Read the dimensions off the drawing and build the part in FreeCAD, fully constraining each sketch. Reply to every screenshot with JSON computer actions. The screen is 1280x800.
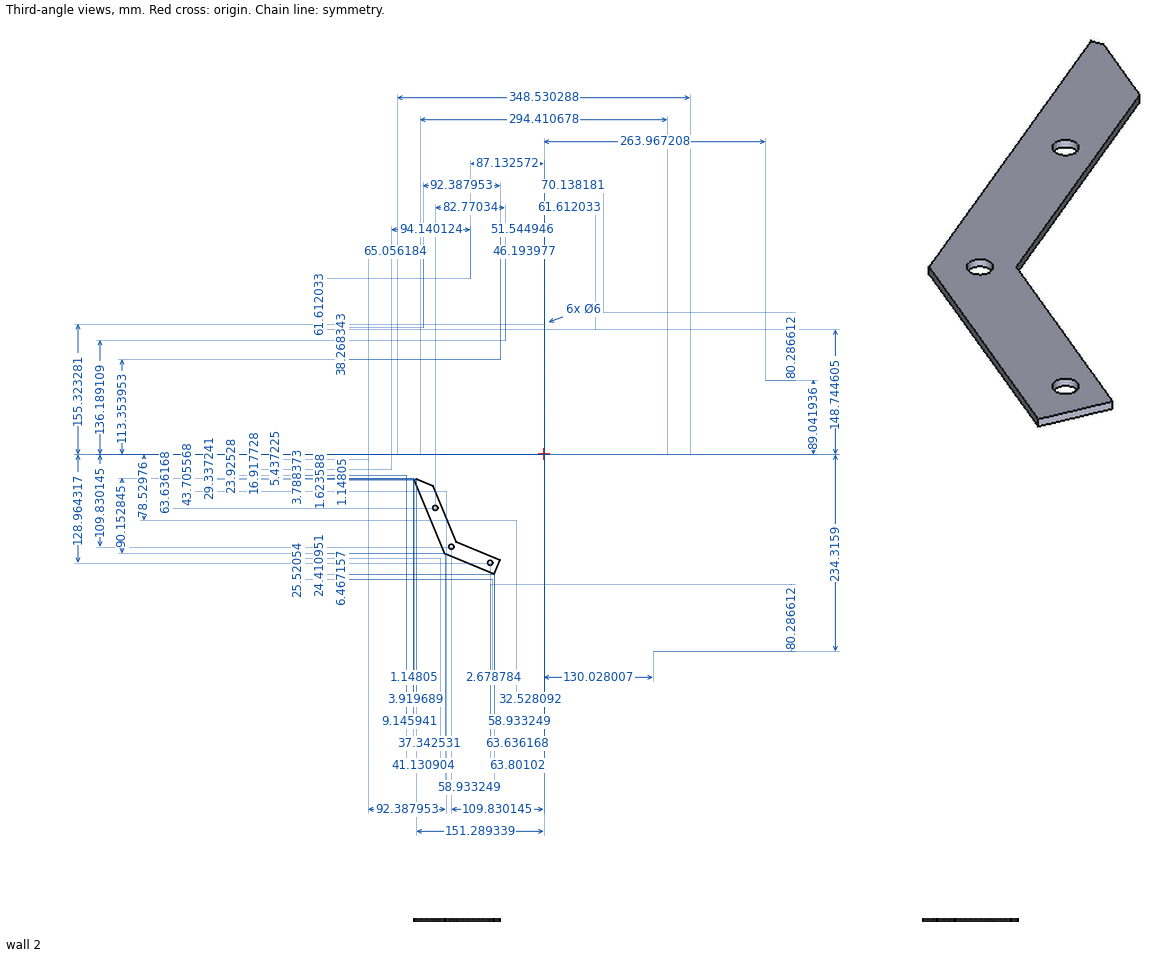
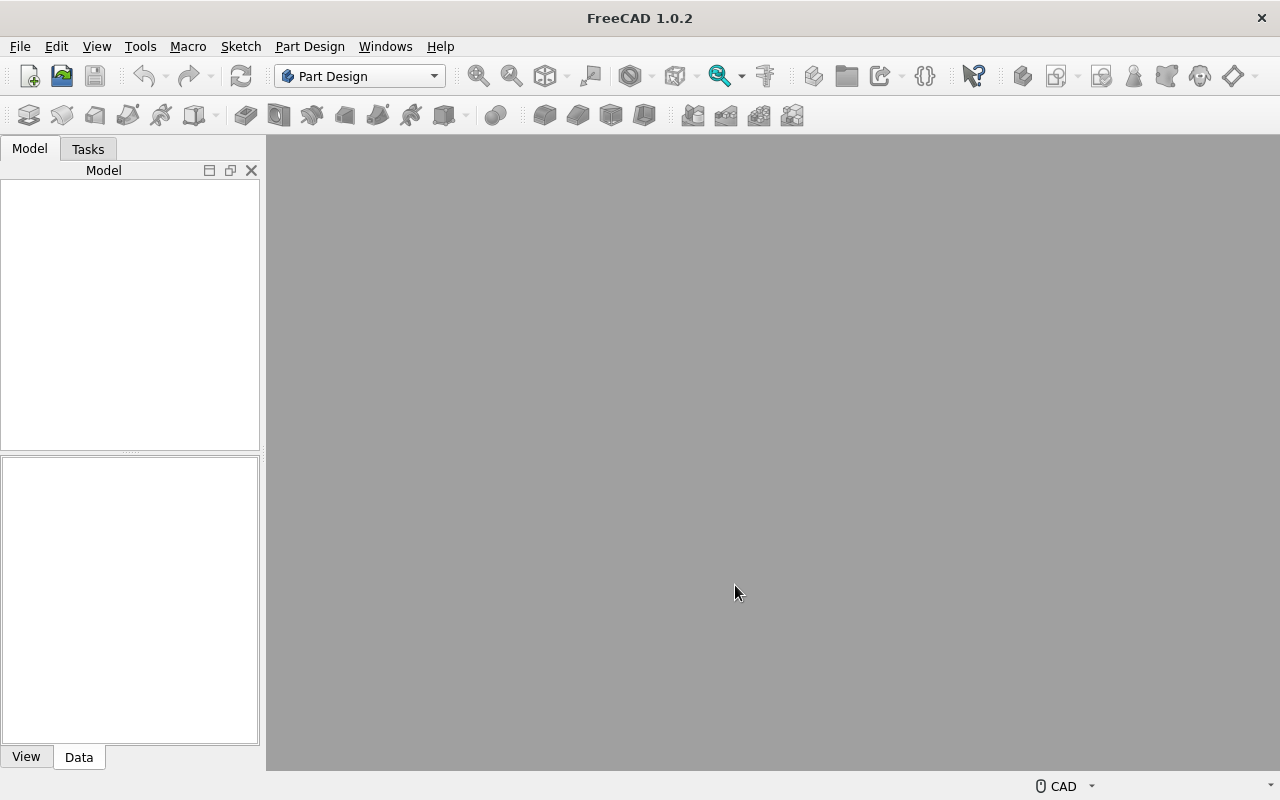
{"action": "left_click", "coordinate": [29, 76]}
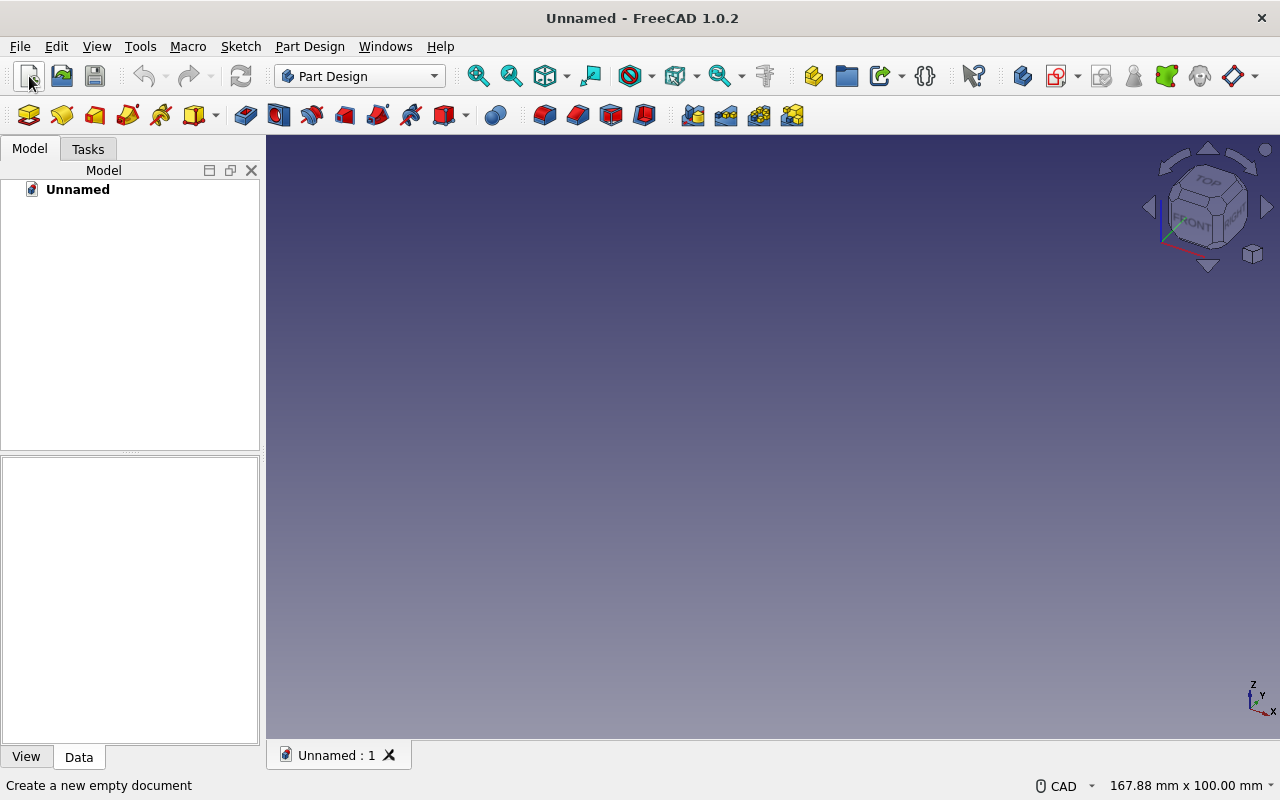
{"action": "left_click", "coordinate": [1056, 76]}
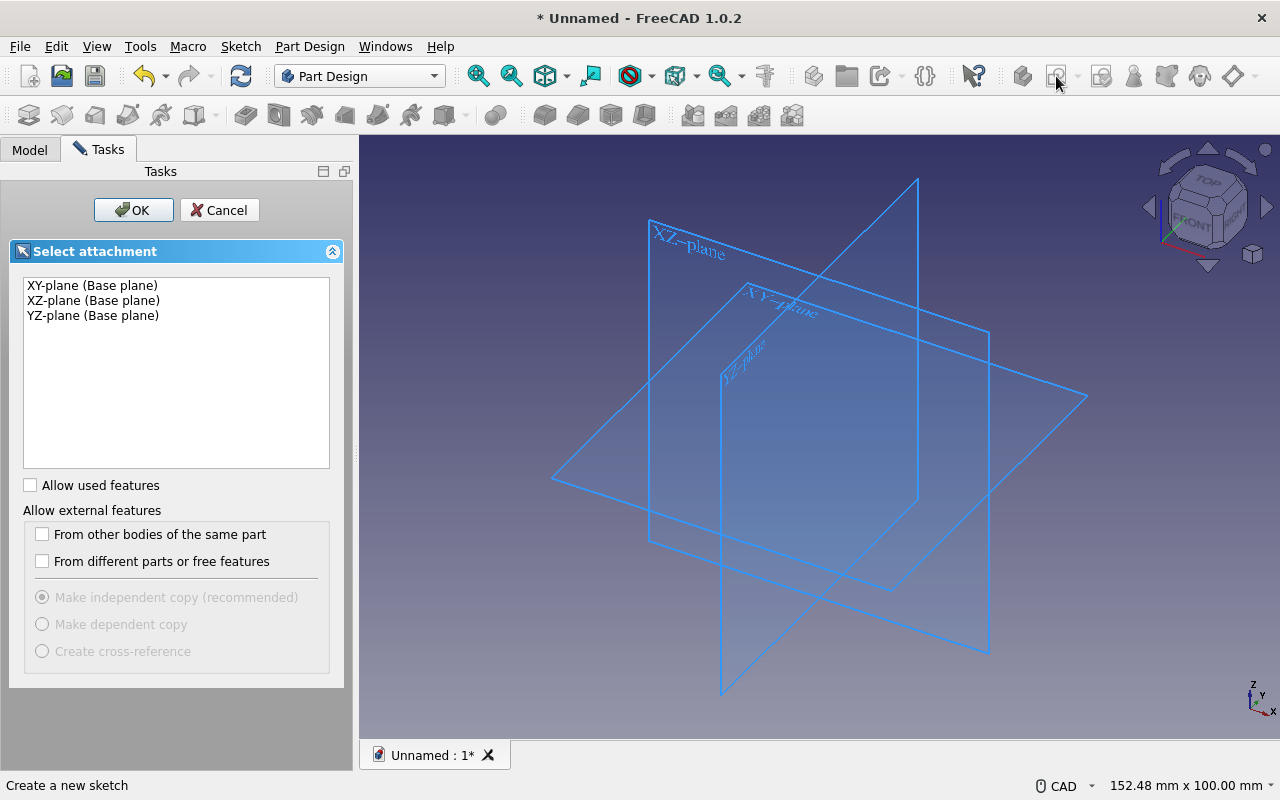
{"action": "left_click", "coordinate": [84, 286]}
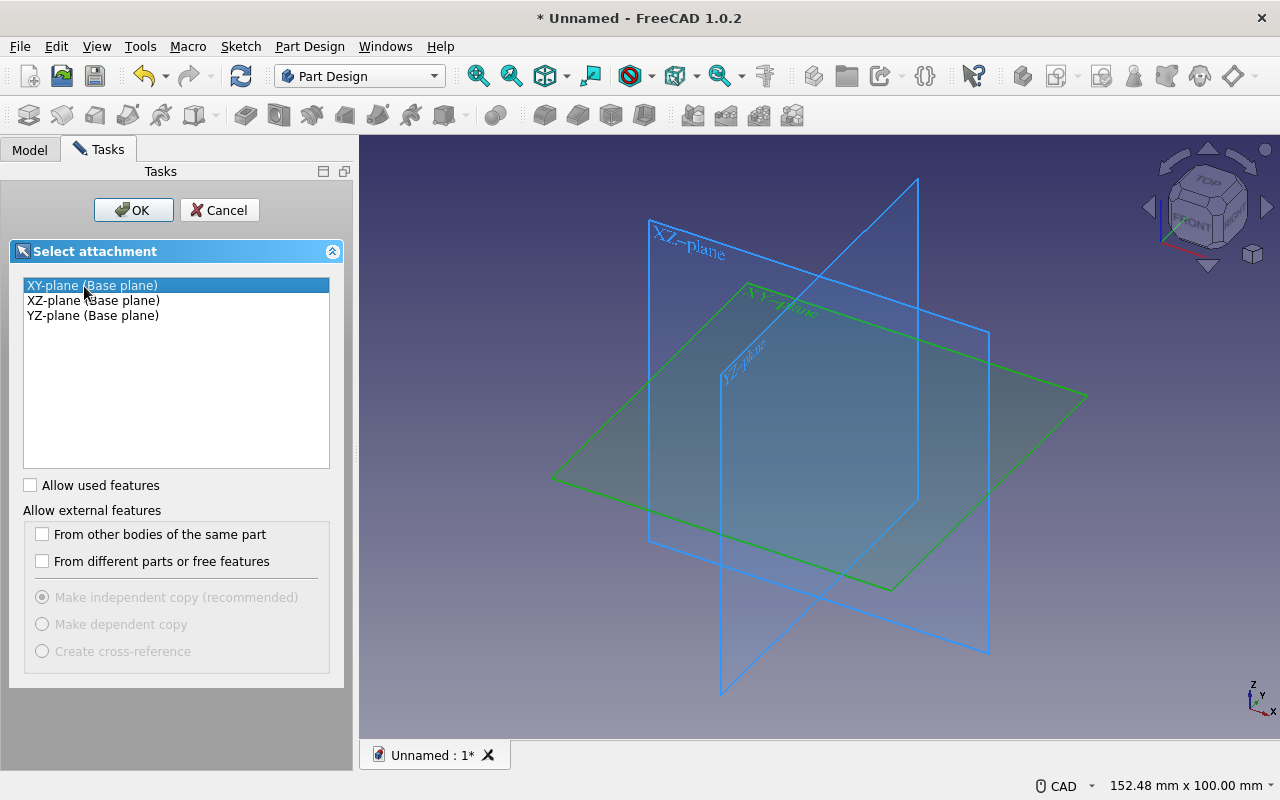
{"action": "left_click", "coordinate": [134, 210]}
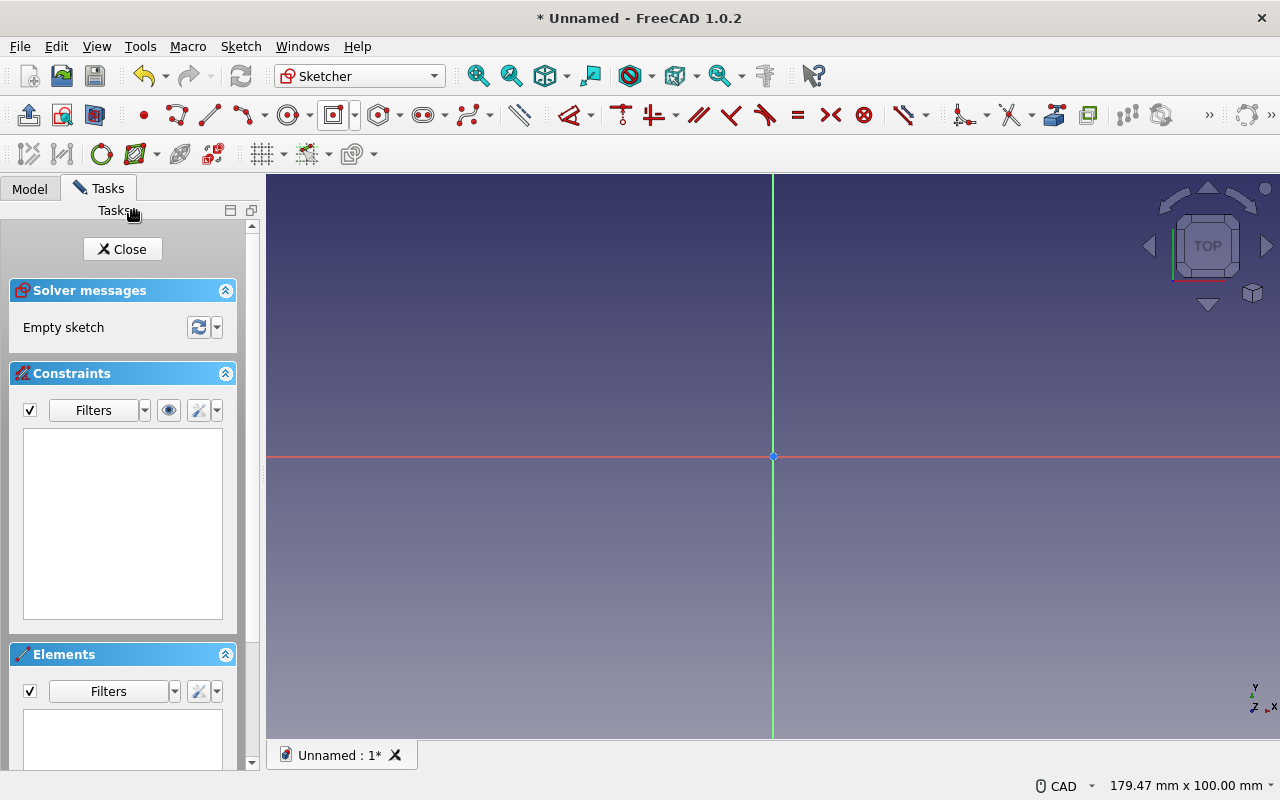
{"action": "scroll", "coordinate": [691, 456], "scroll_direction": "down", "scroll_amount": 9}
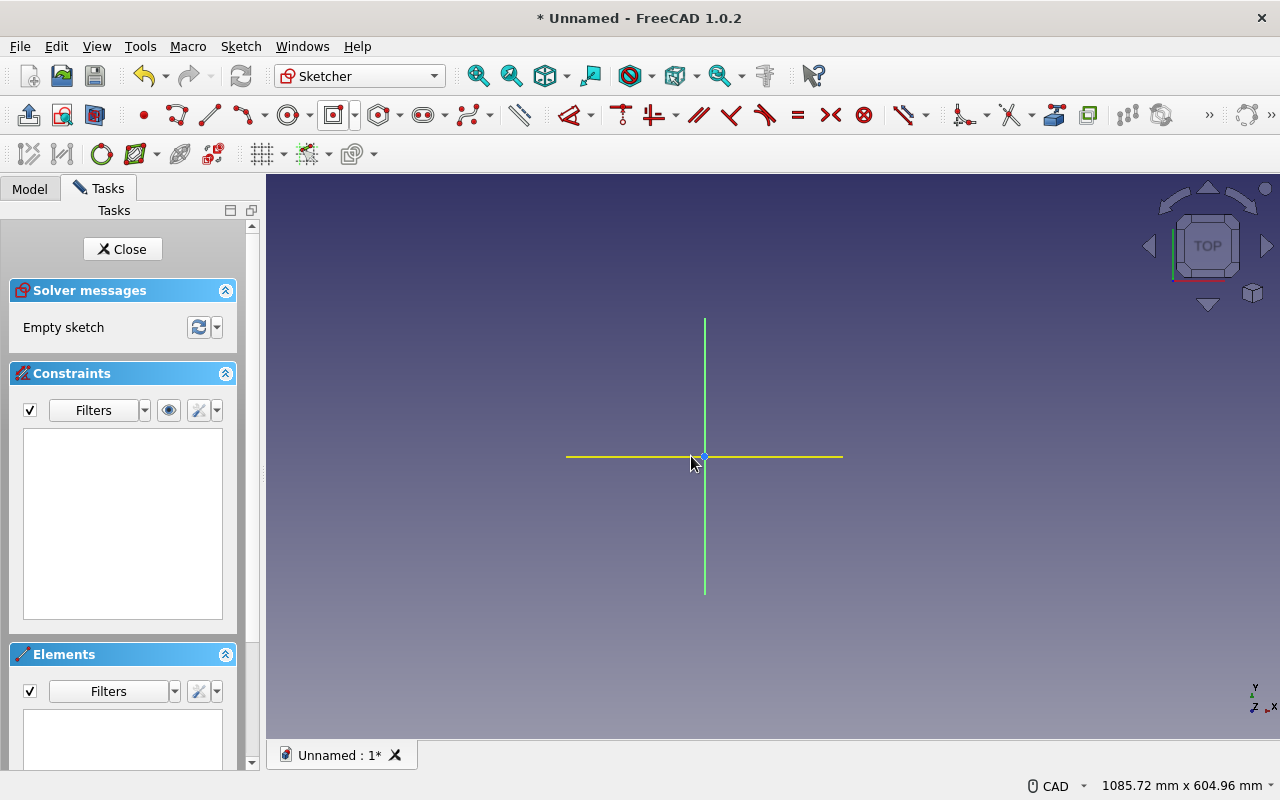
{"action": "key", "text": "g p 8"}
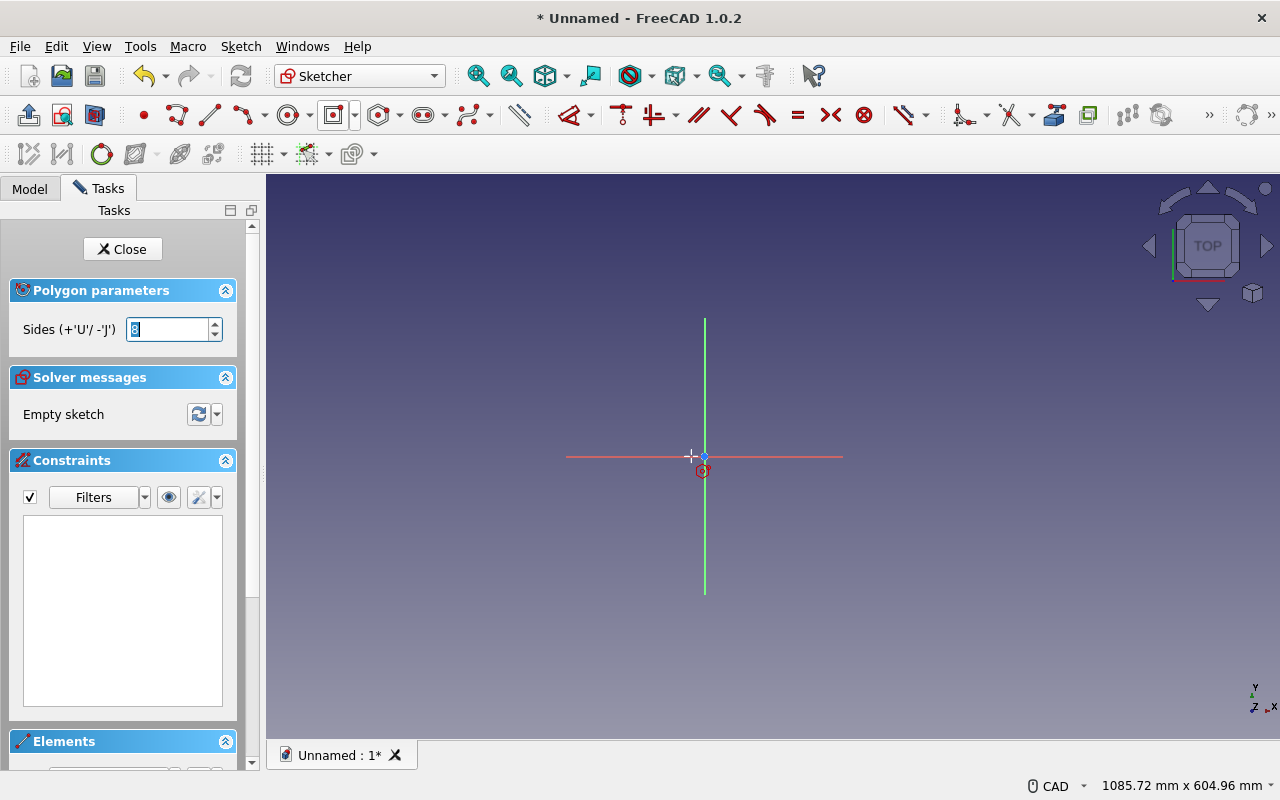
{"action": "left_click", "coordinate": [705, 456]}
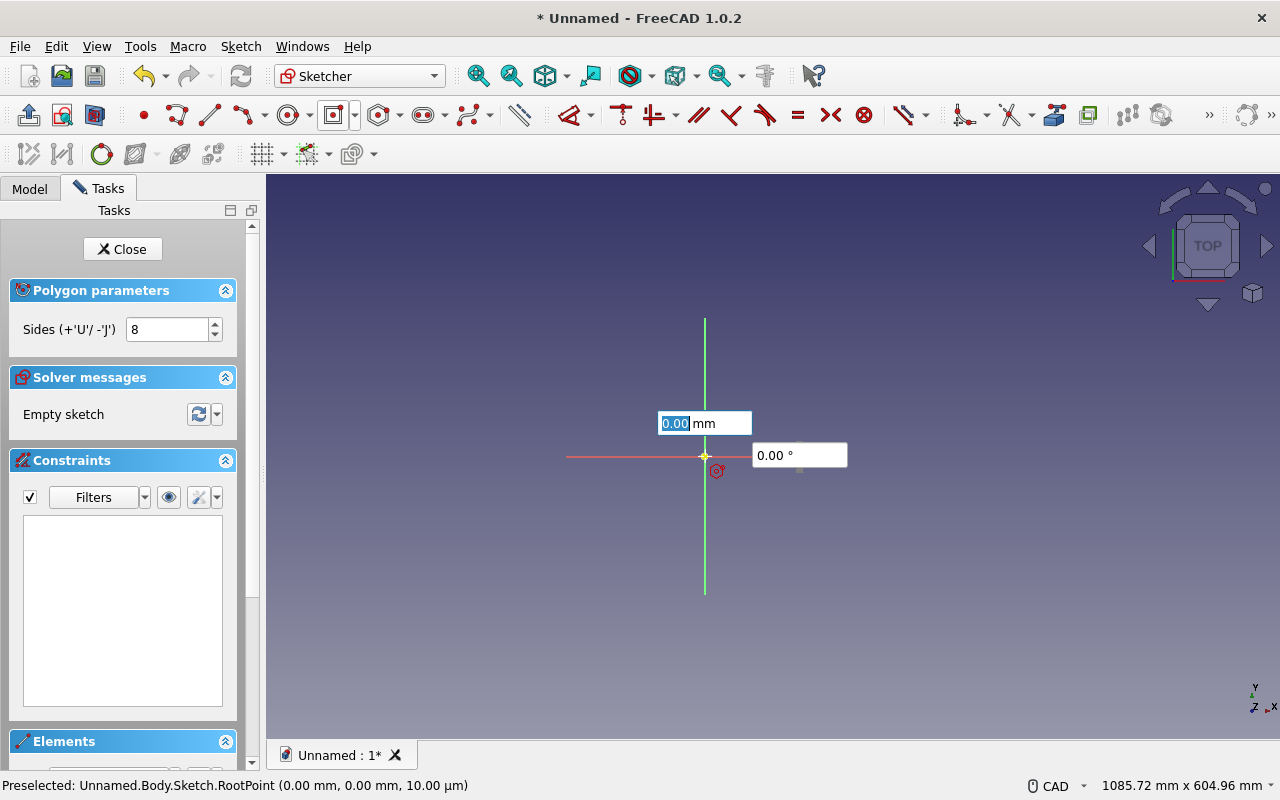
{"action": "left_click", "coordinate": [542, 456]}
{"action": "right_click", "coordinate": [542, 456]}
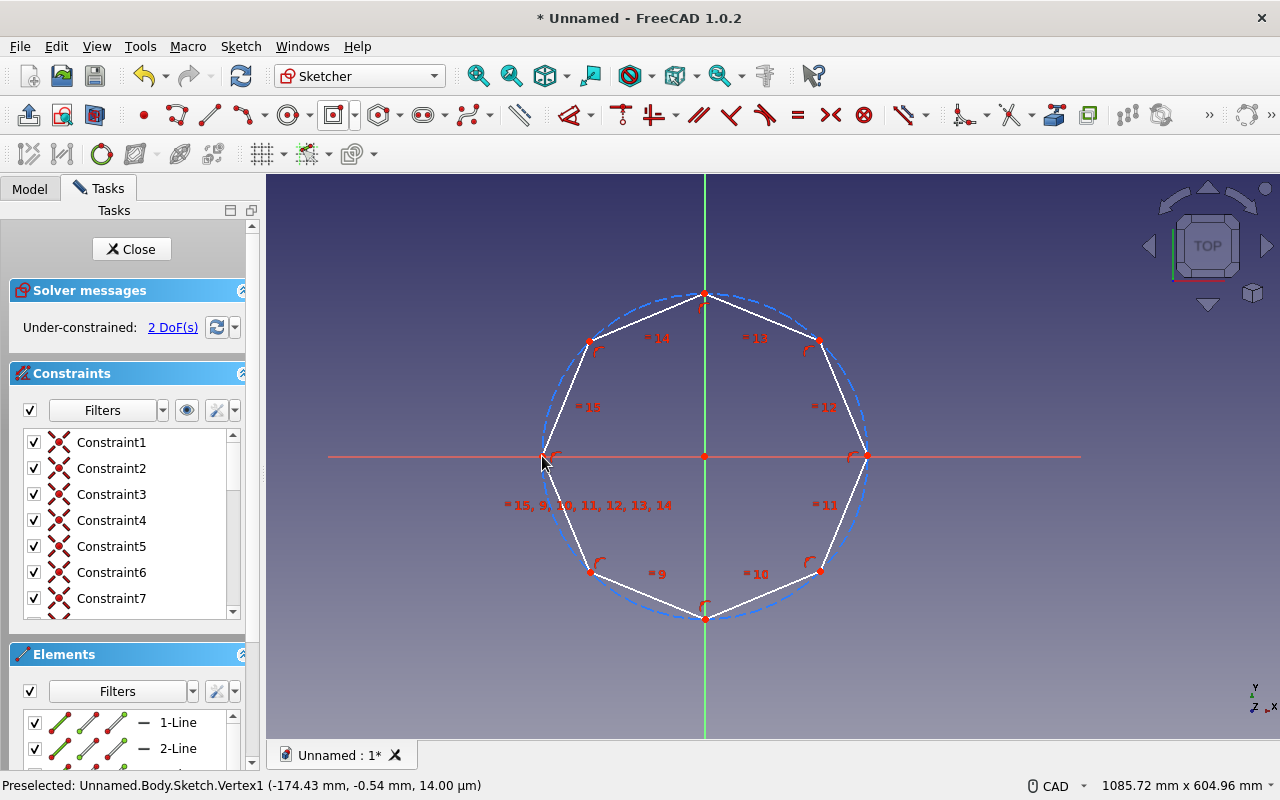
{"action": "left_click", "coordinate": [542, 457]}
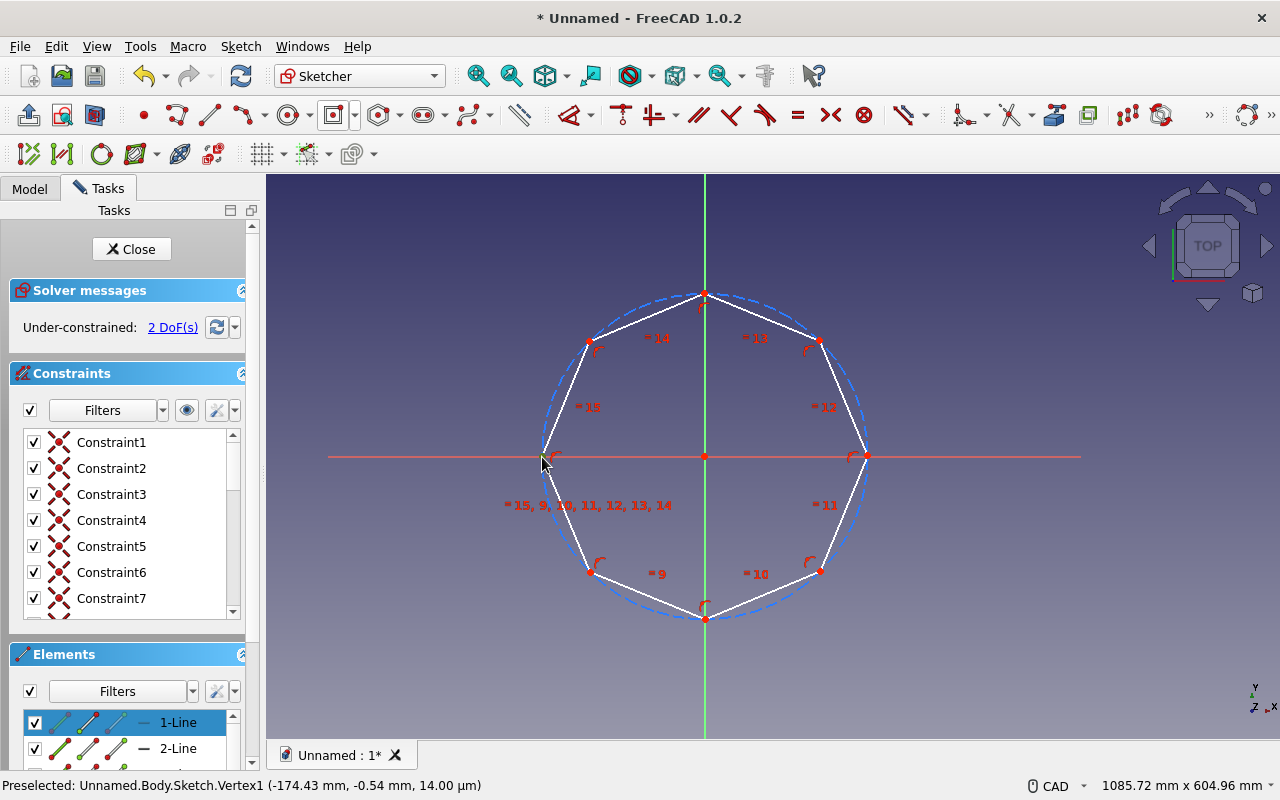
{"action": "left_click", "coordinate": [353, 456]}